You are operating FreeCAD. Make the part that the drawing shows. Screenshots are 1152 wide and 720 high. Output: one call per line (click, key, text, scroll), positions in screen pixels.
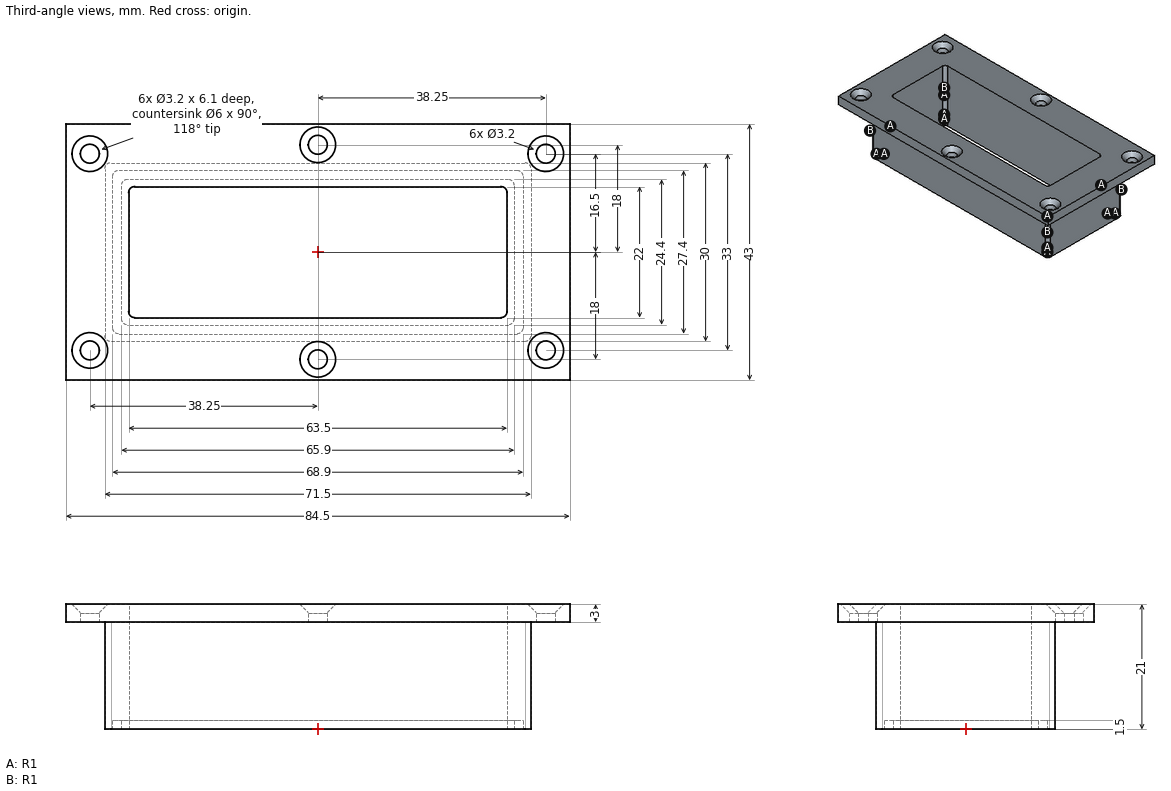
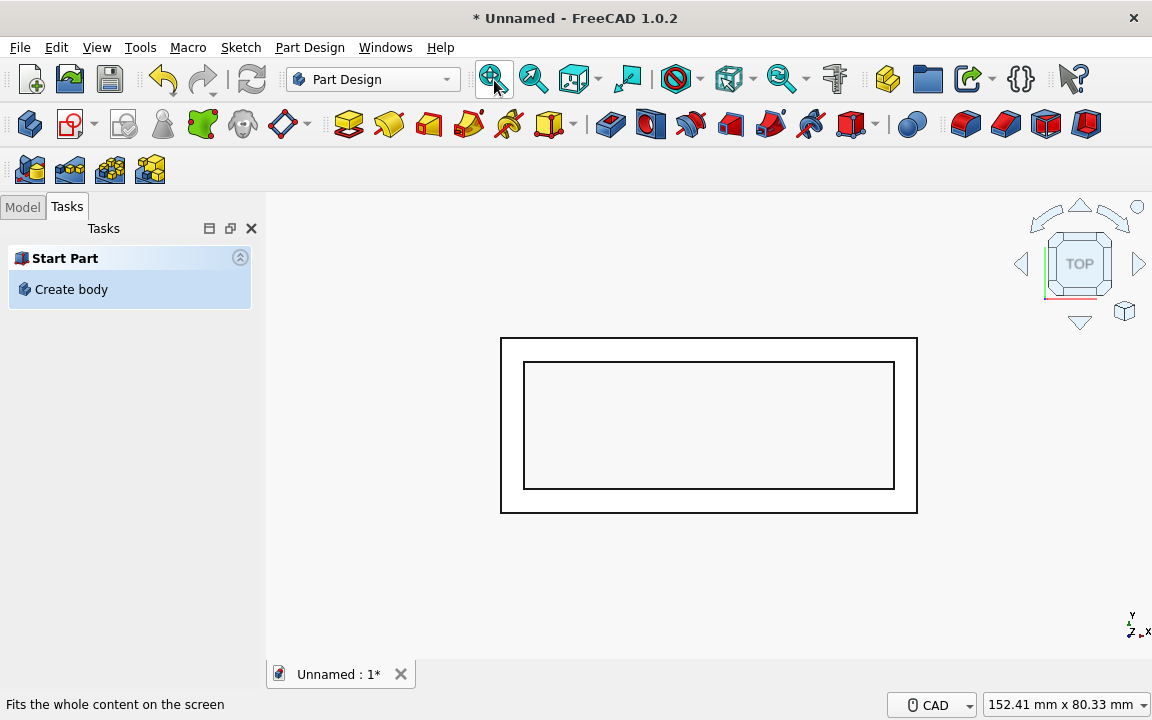
click(887, 350)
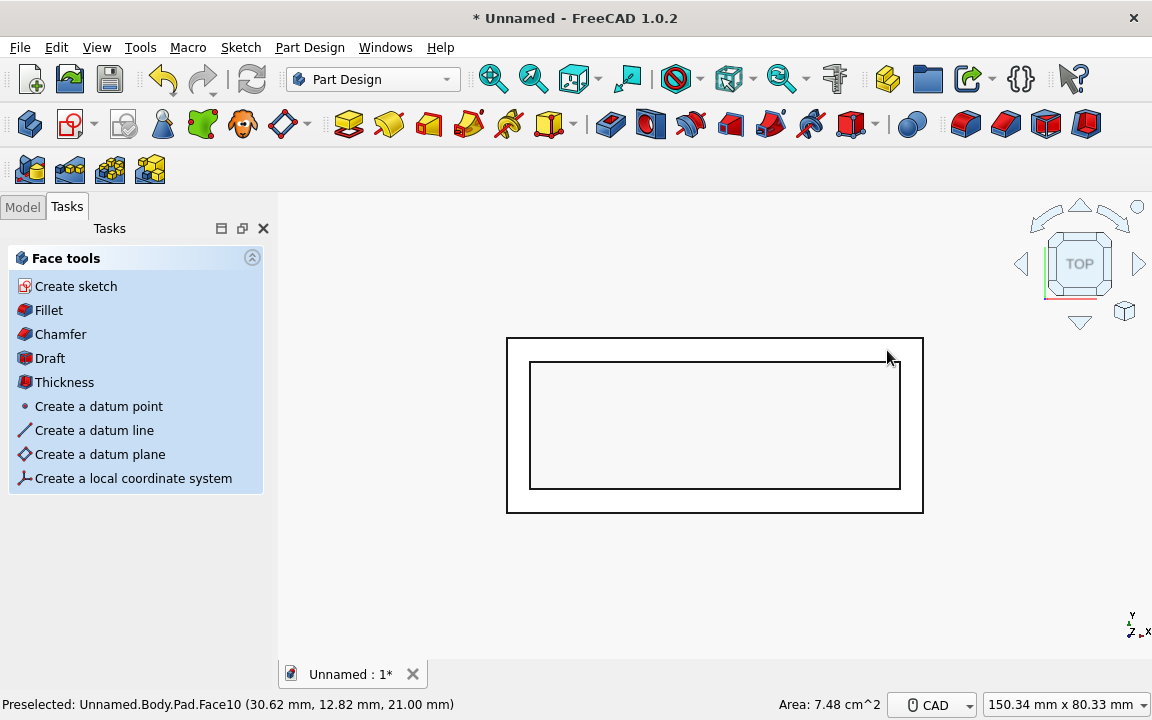
click(70, 124)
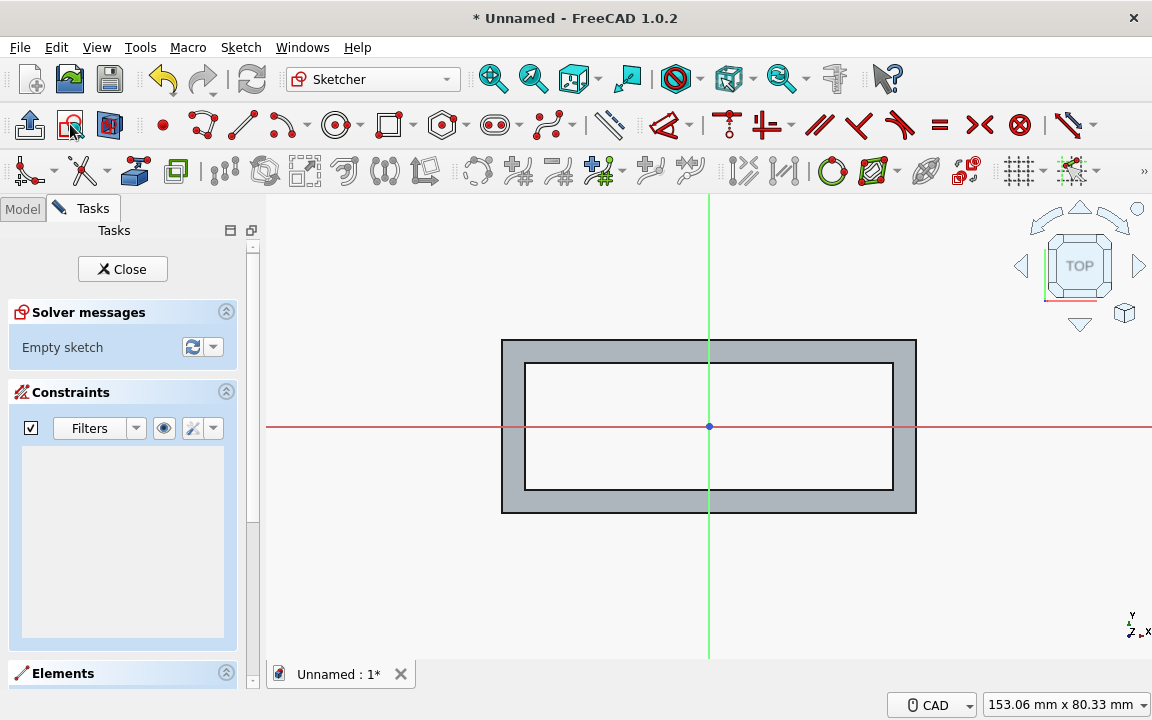
key(g)
key(v)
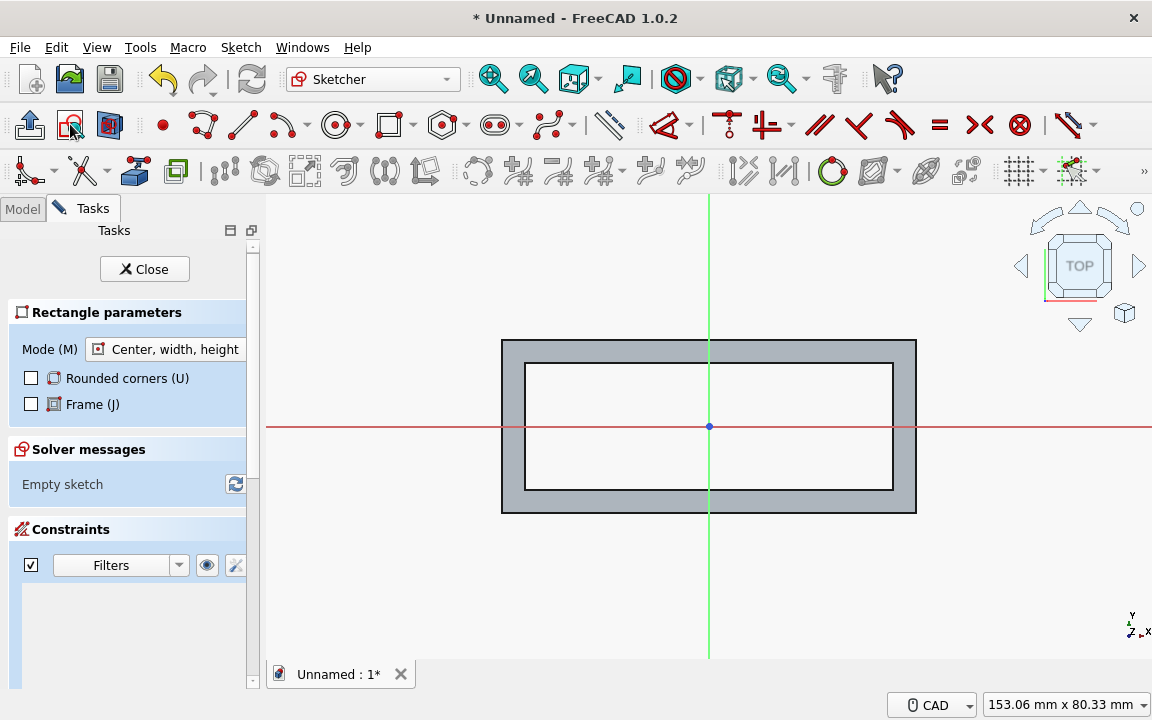
click(709, 426)
click(954, 302)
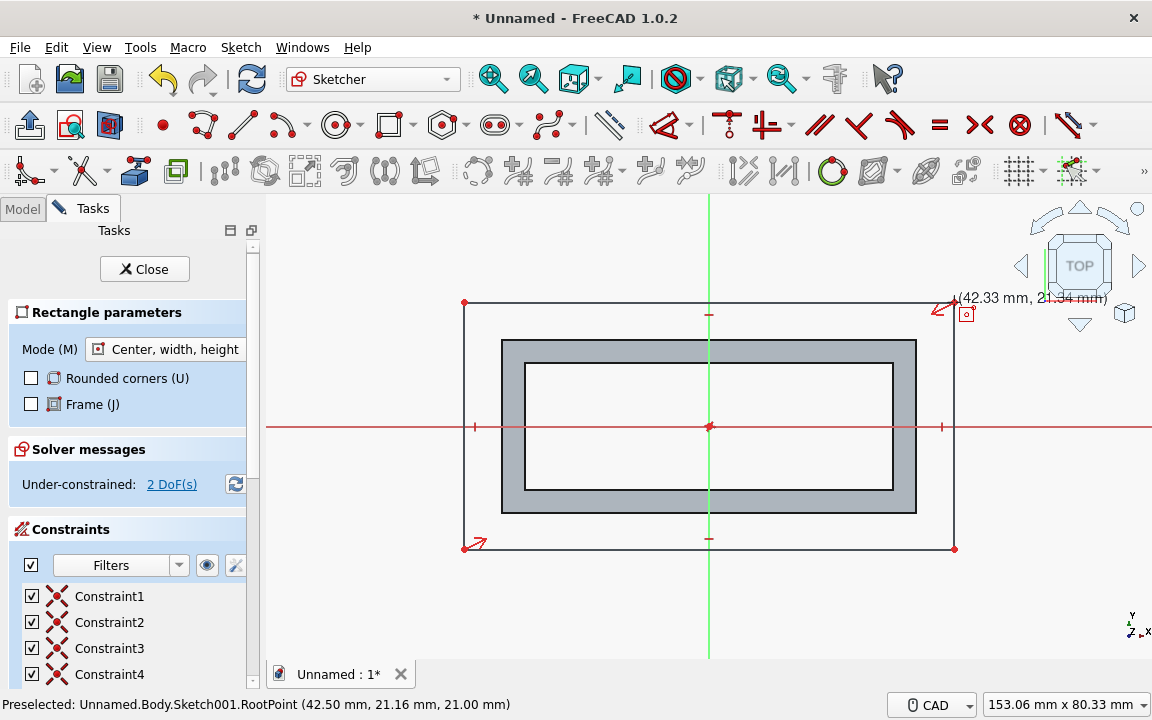
click(709, 426)
click(916, 340)
key(Escape)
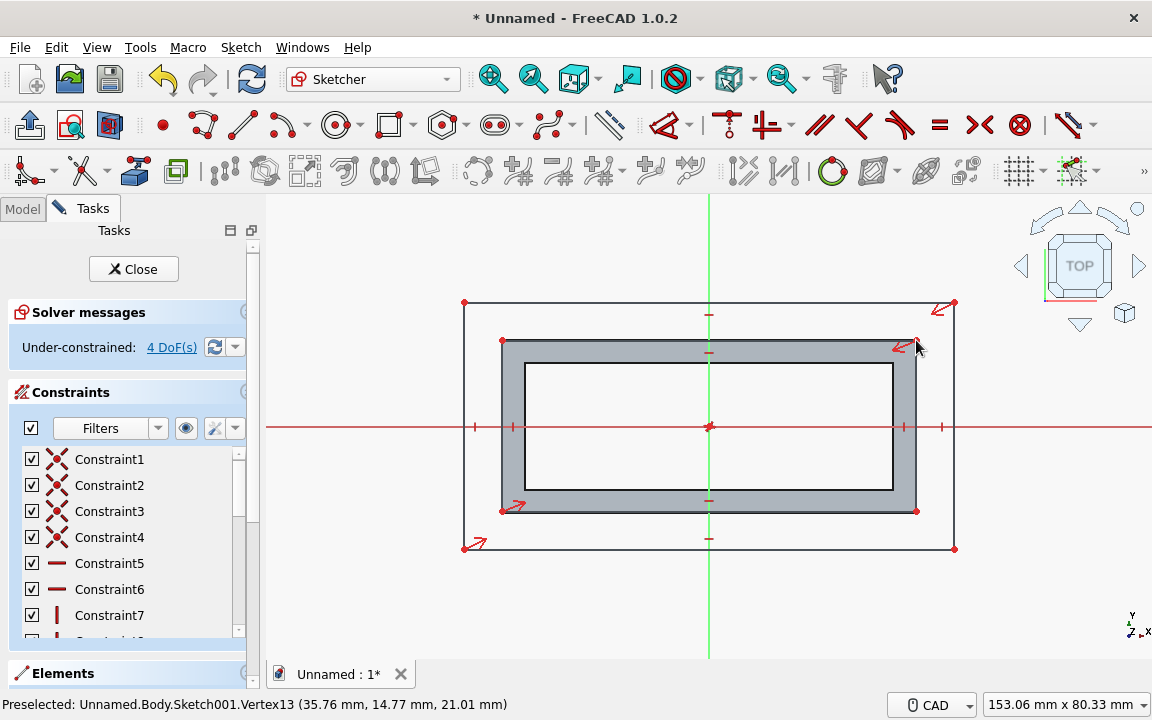
click(664, 126)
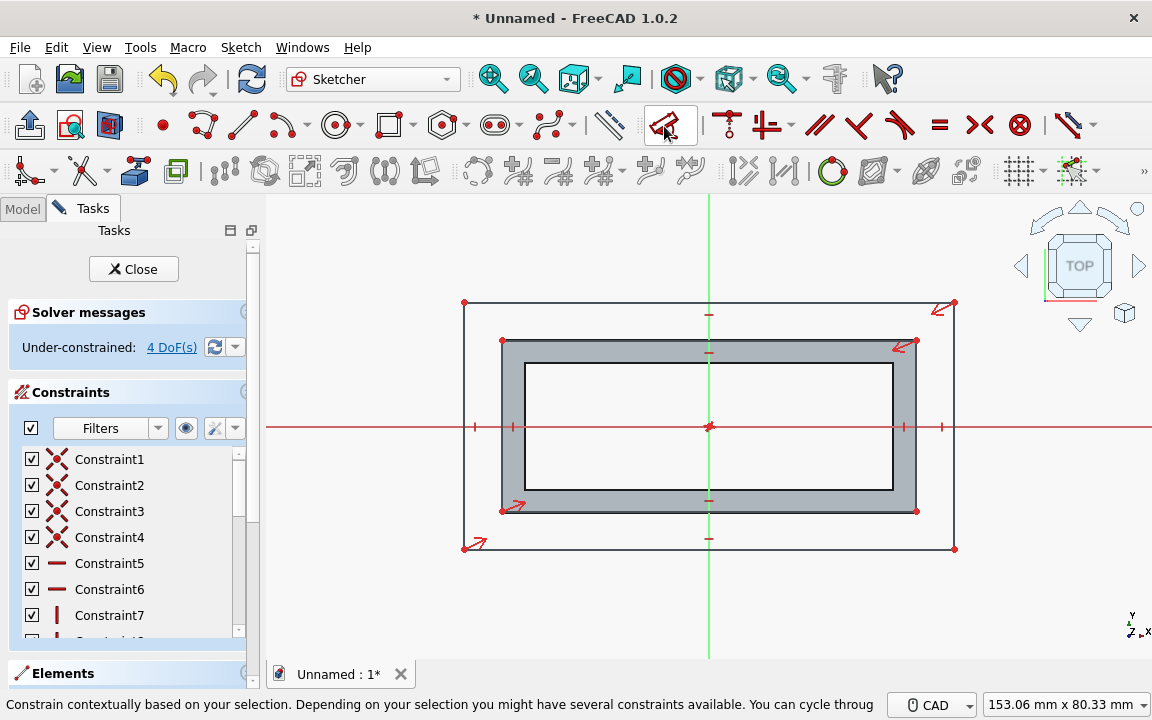
click(954, 476)
click(896, 370)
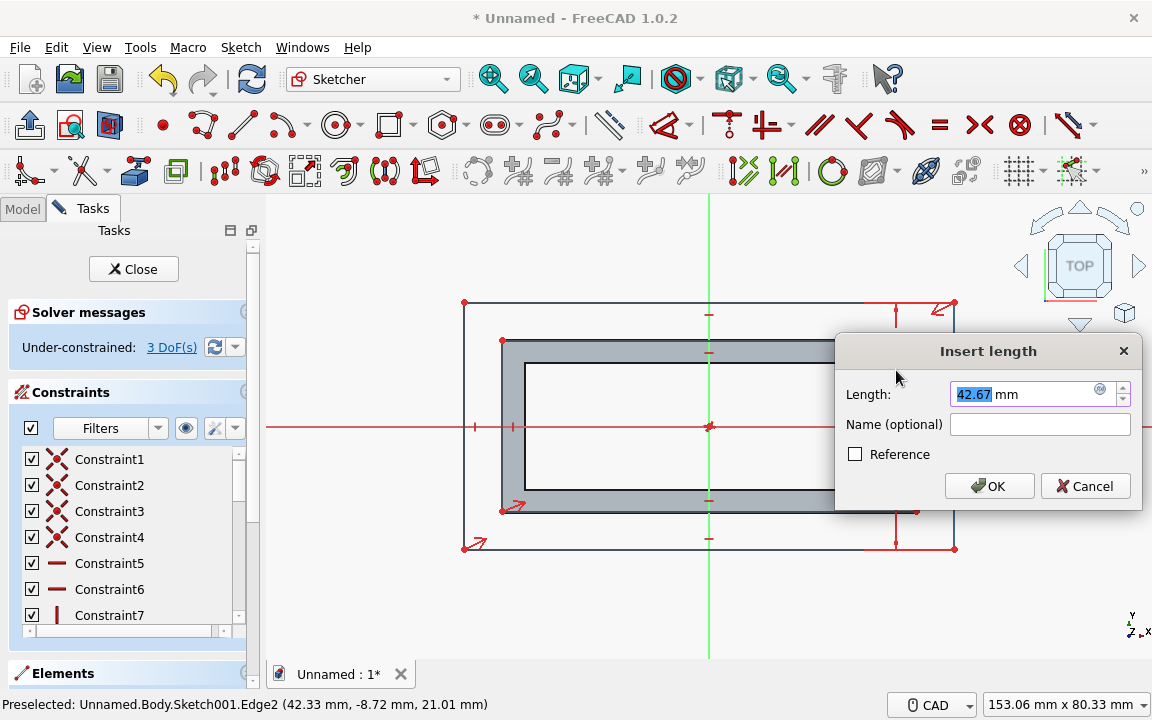
text(43)
key(Return)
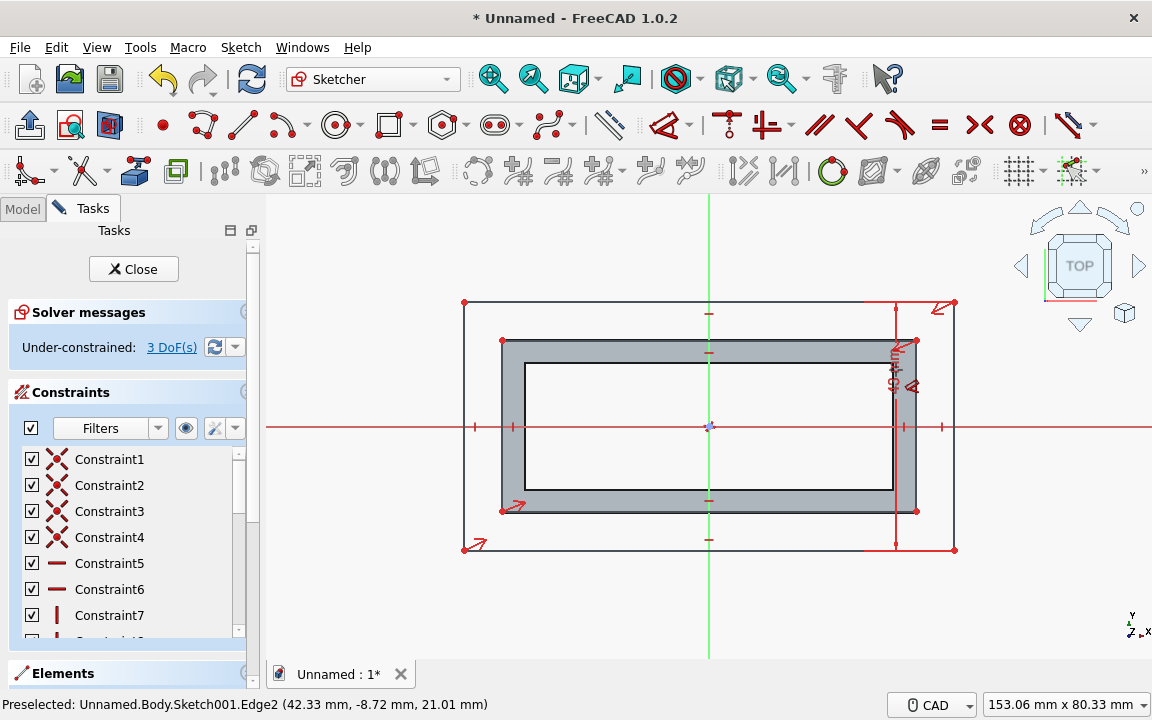
click(916, 461)
click(882, 466)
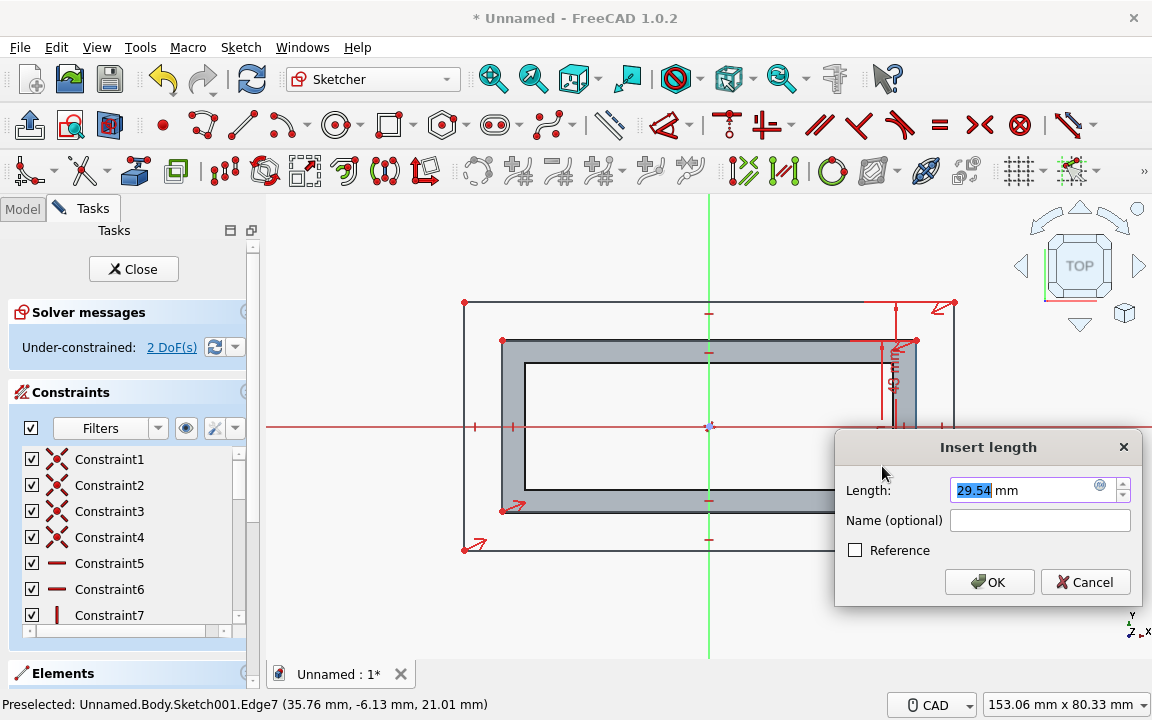
text(30)
key(Return)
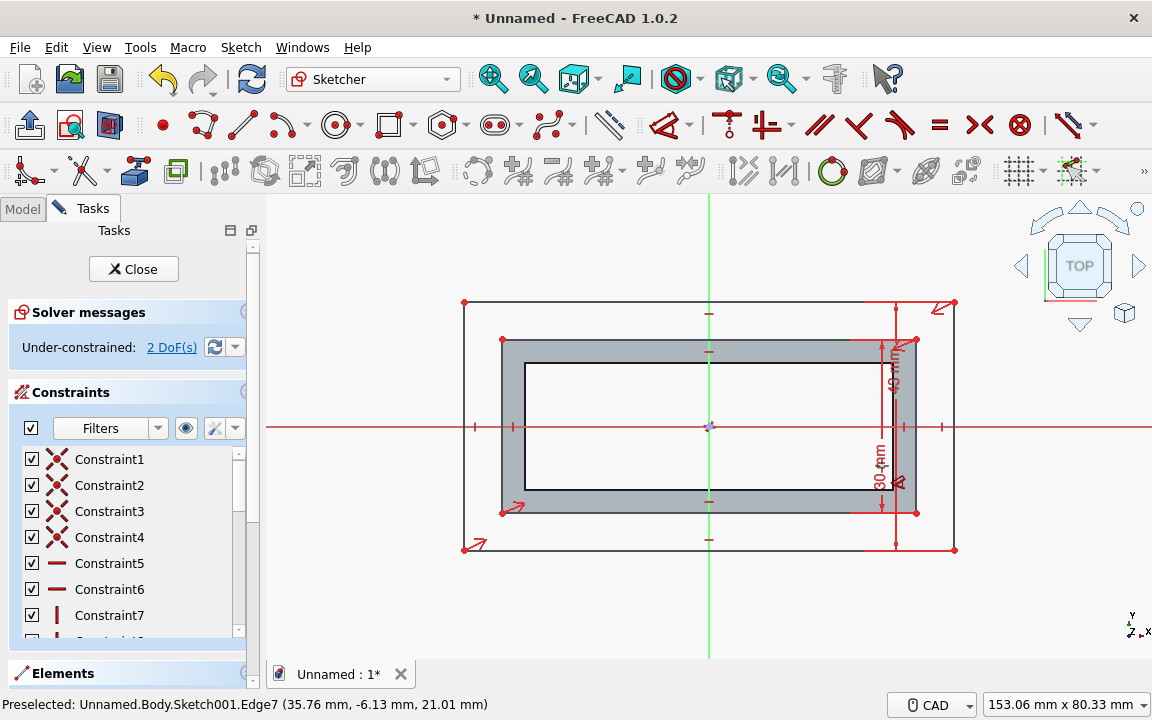
click(611, 551)
click(596, 585)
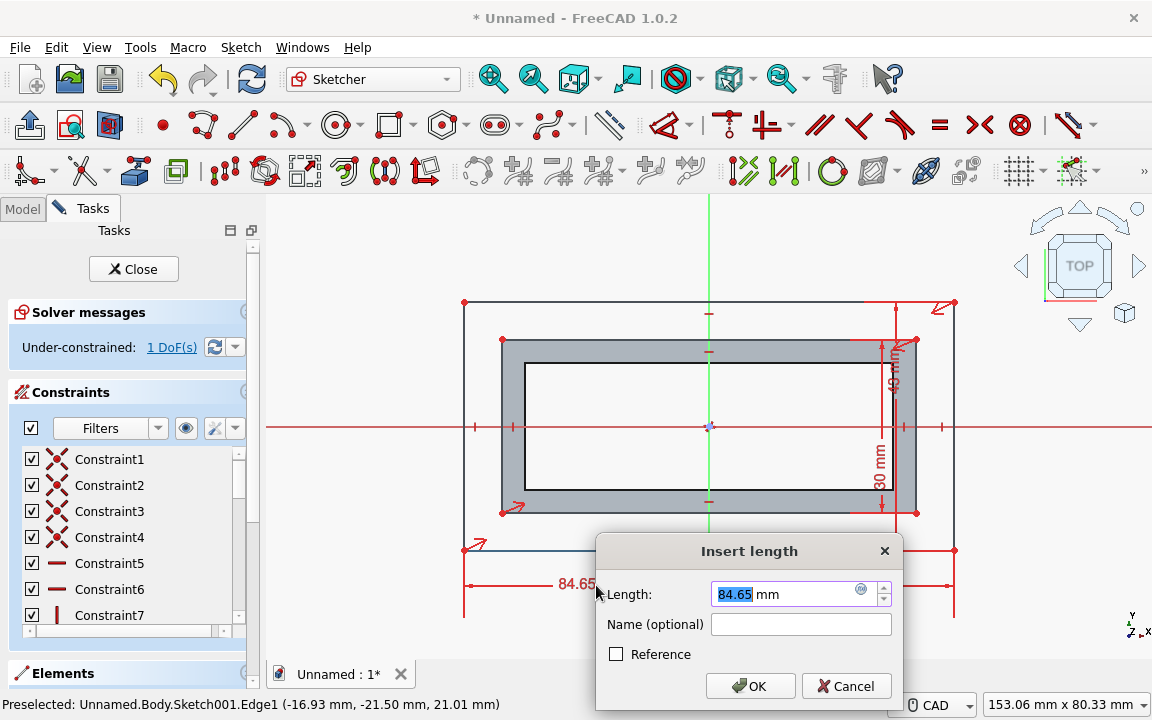
text(84.5)
key(Return)